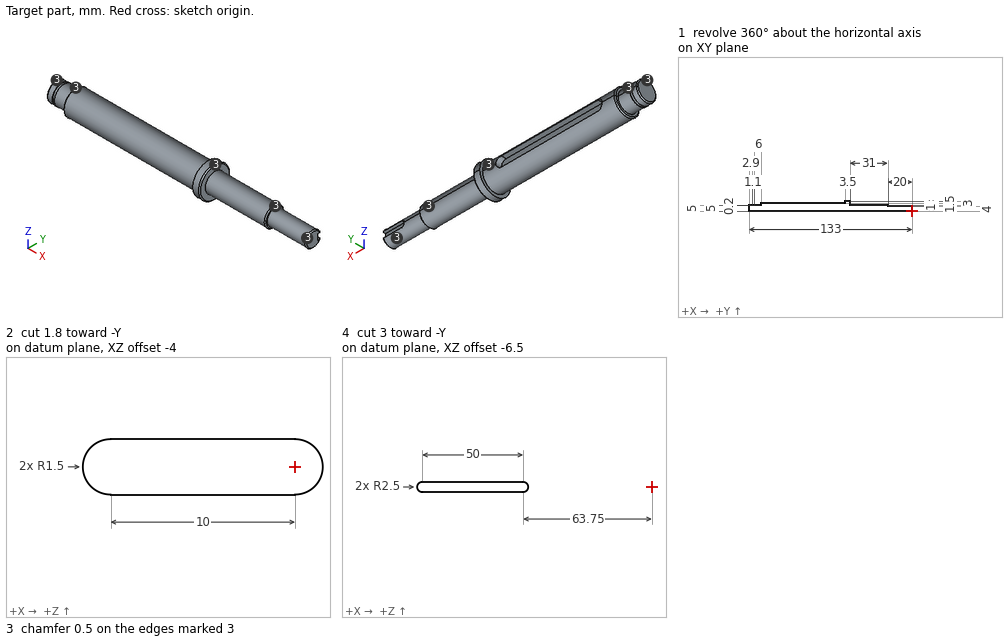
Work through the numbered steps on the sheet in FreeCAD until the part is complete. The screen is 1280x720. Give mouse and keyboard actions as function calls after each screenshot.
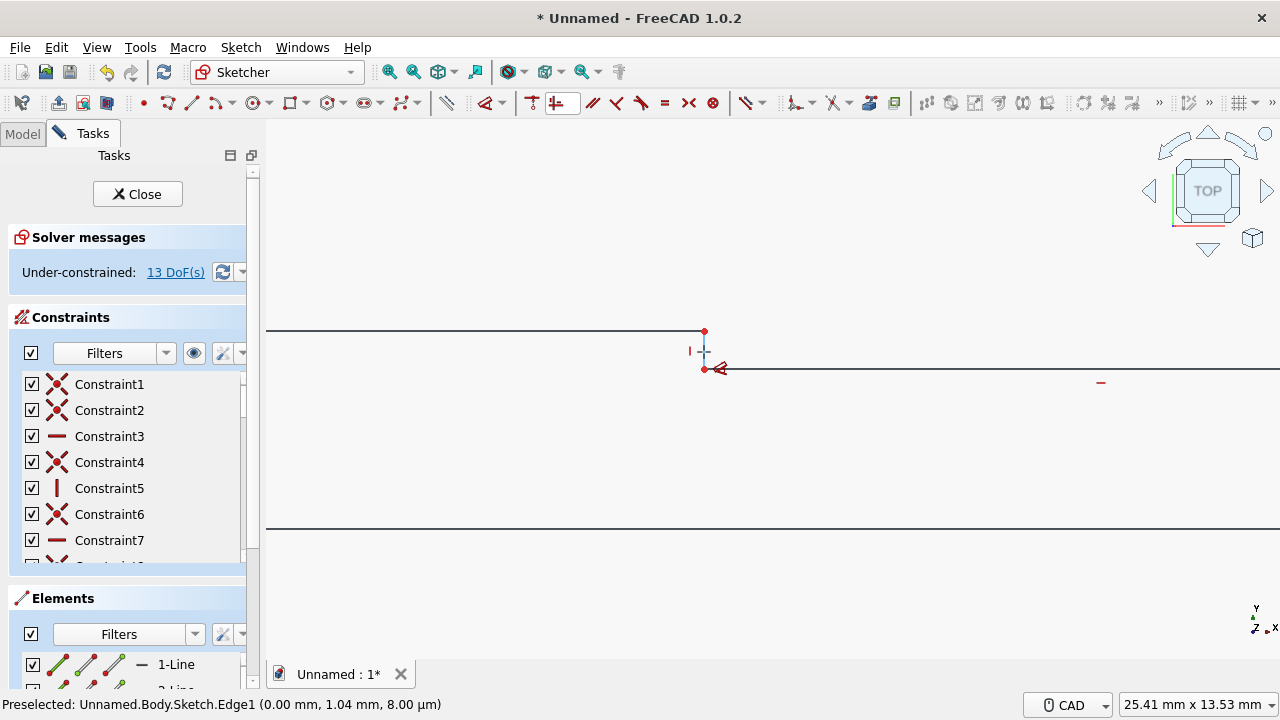
click(704, 350)
click(738, 350)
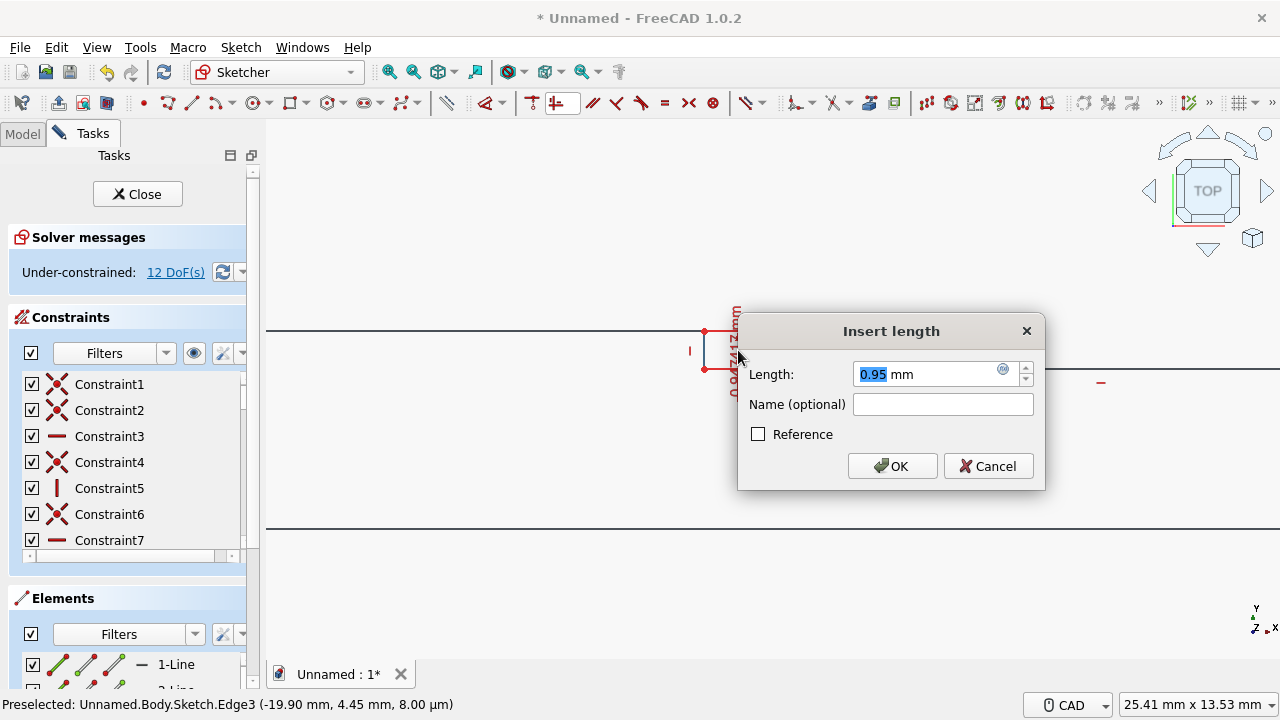
text(1)
key(Return)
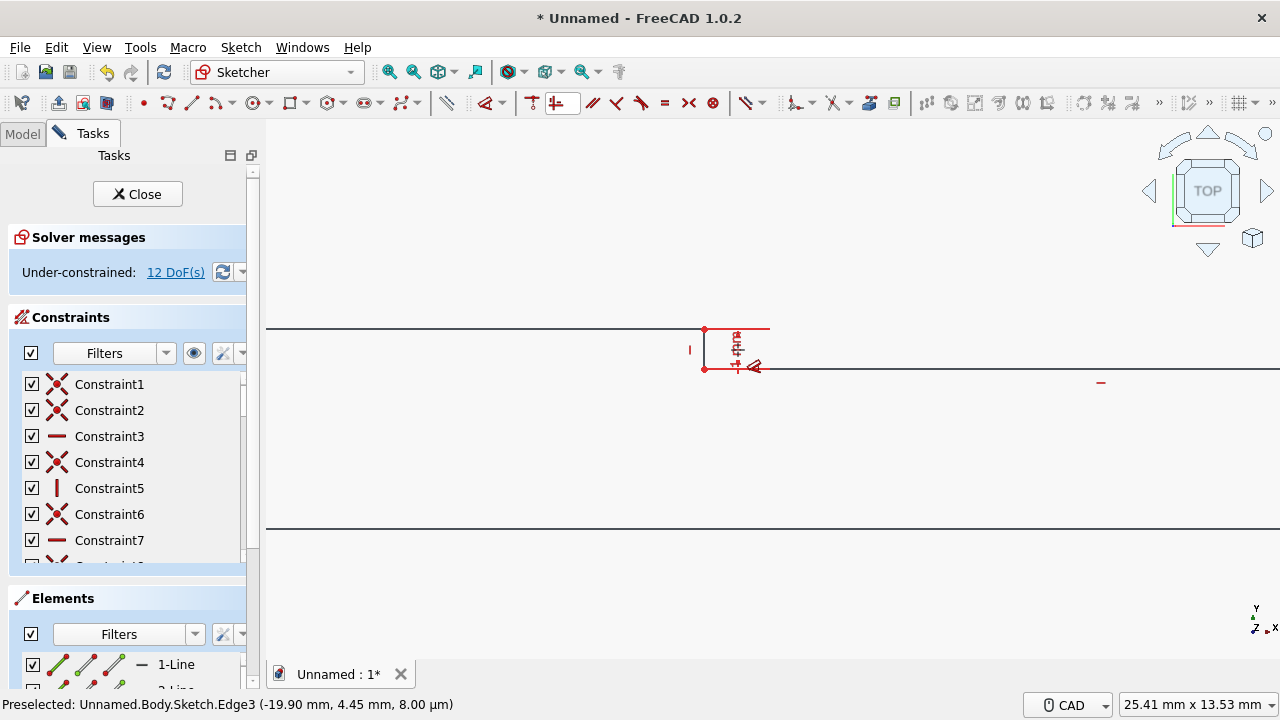
scroll(936, 391, down, 11)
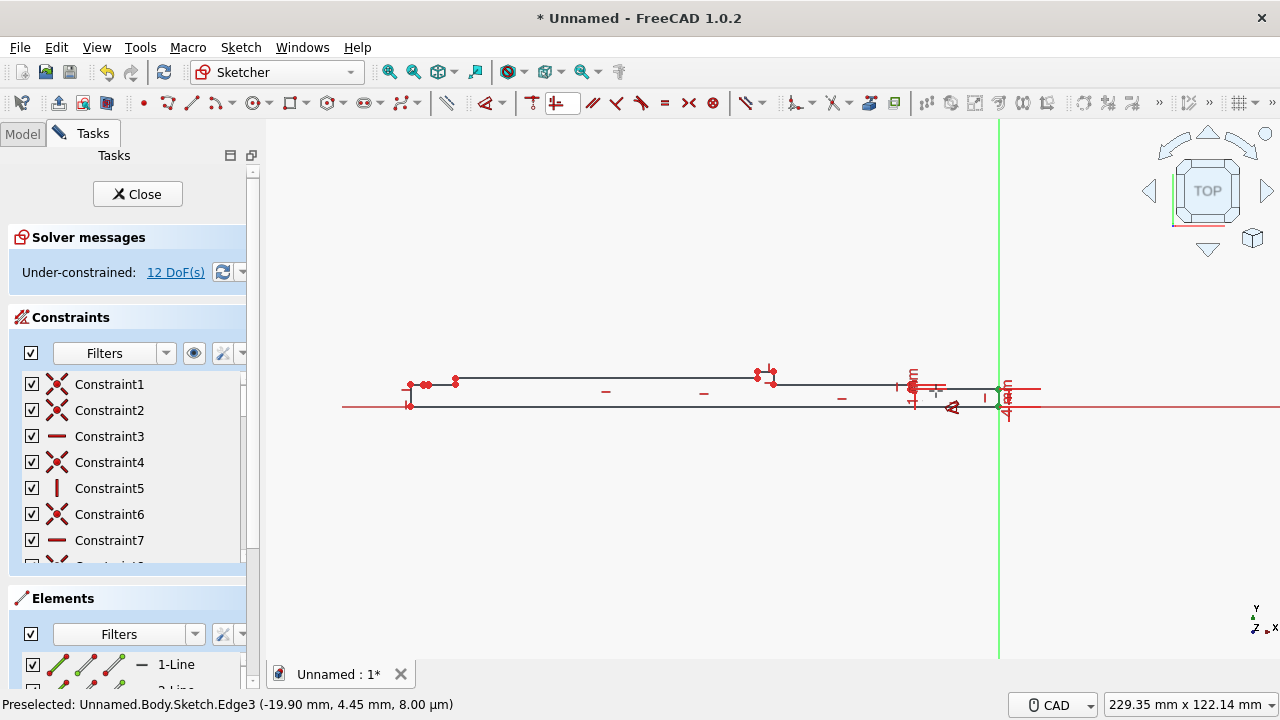
scroll(774, 381, up, 7)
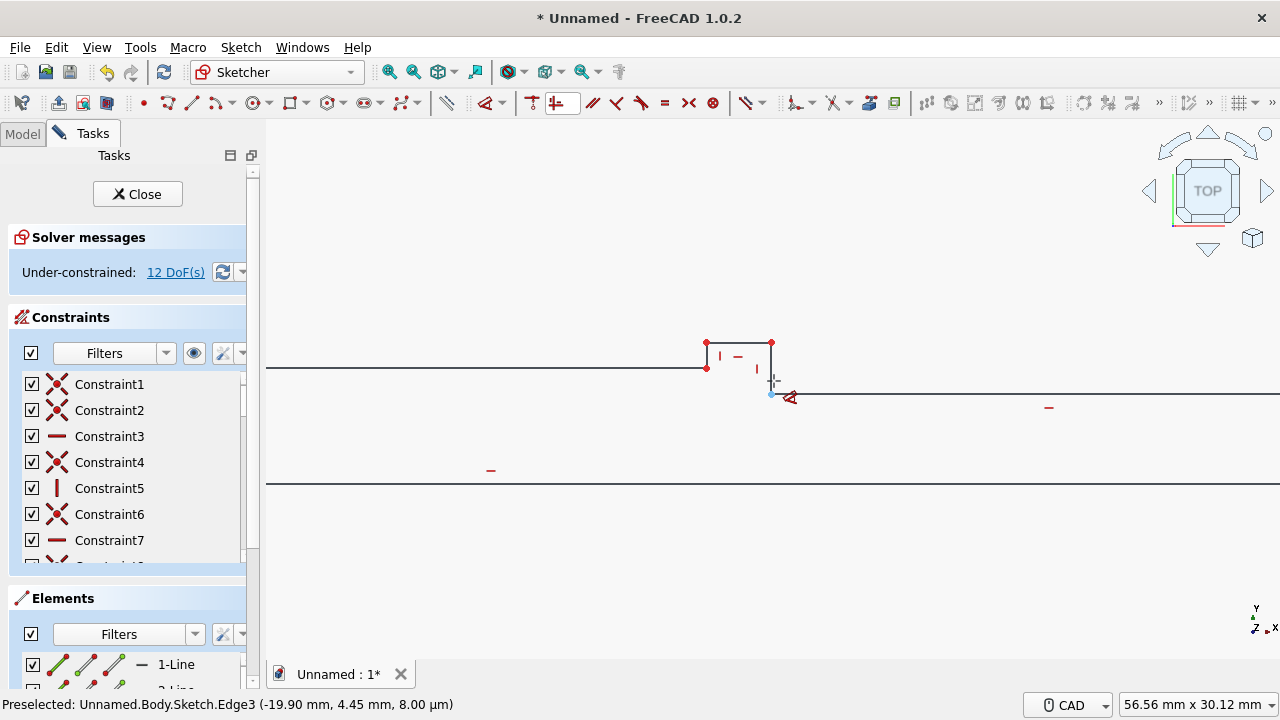
click(771, 379)
click(805, 368)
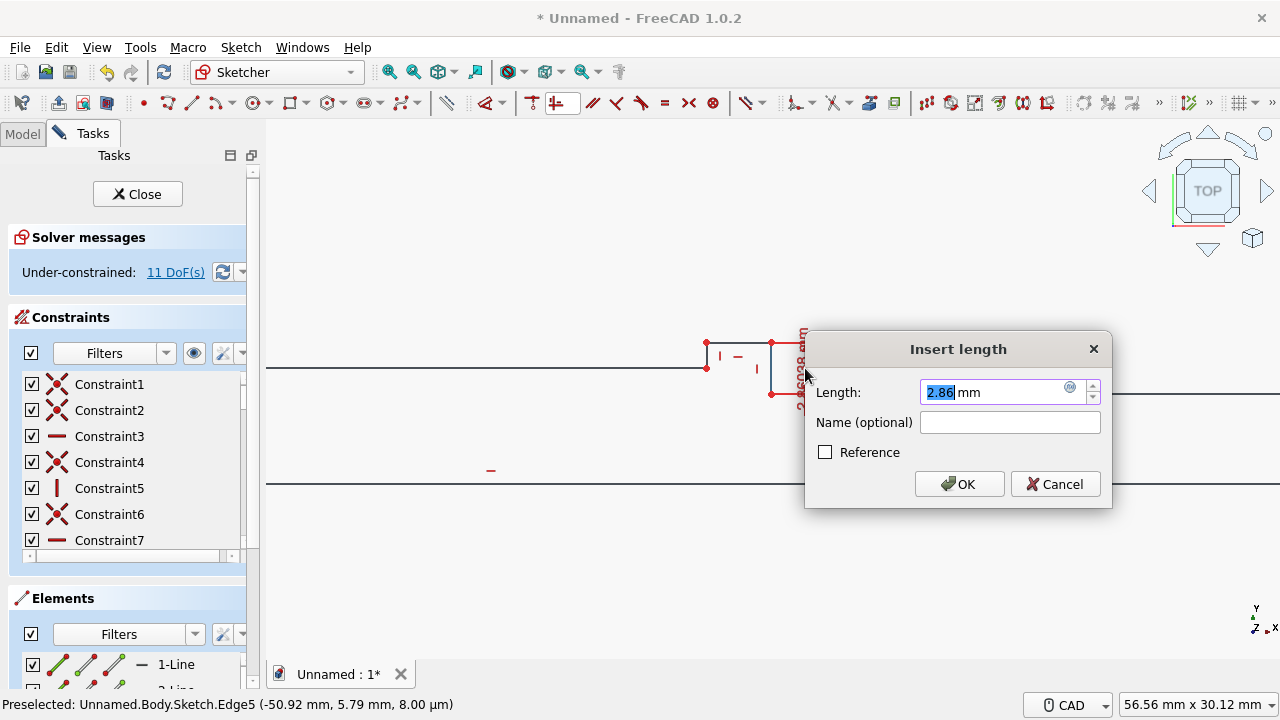
text(3)
key(Return)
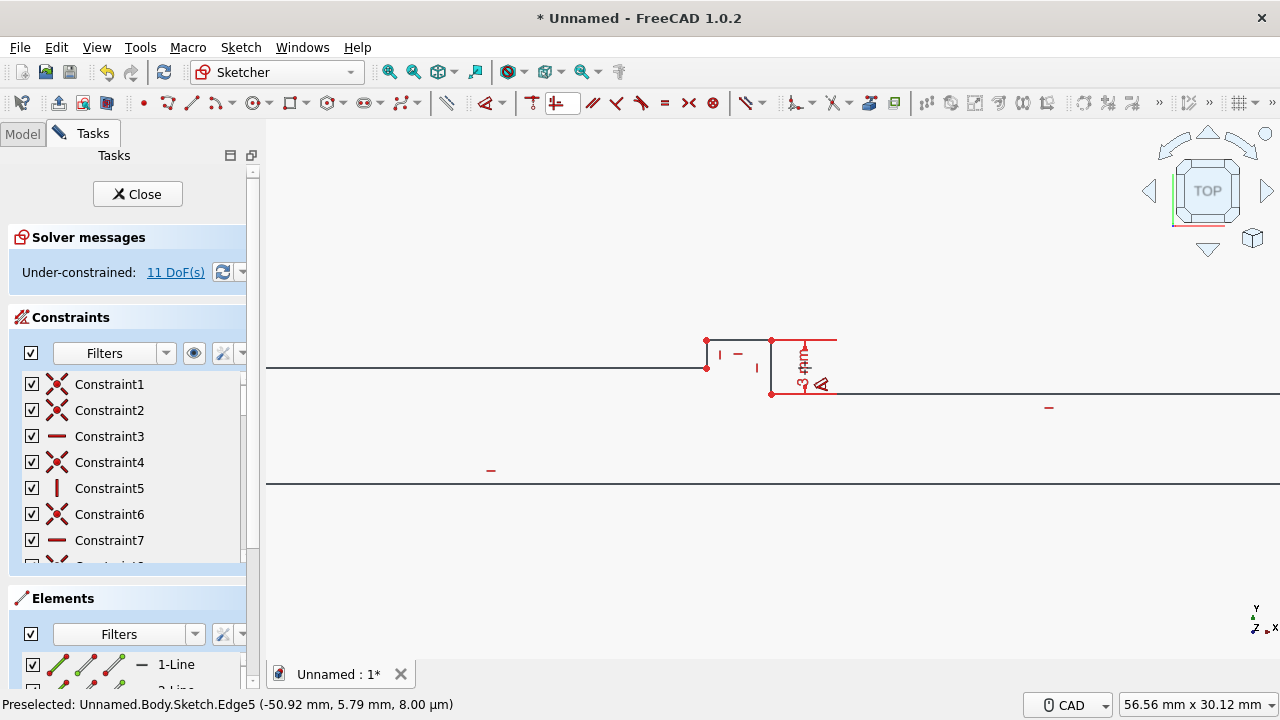
scroll(774, 381, down, 7)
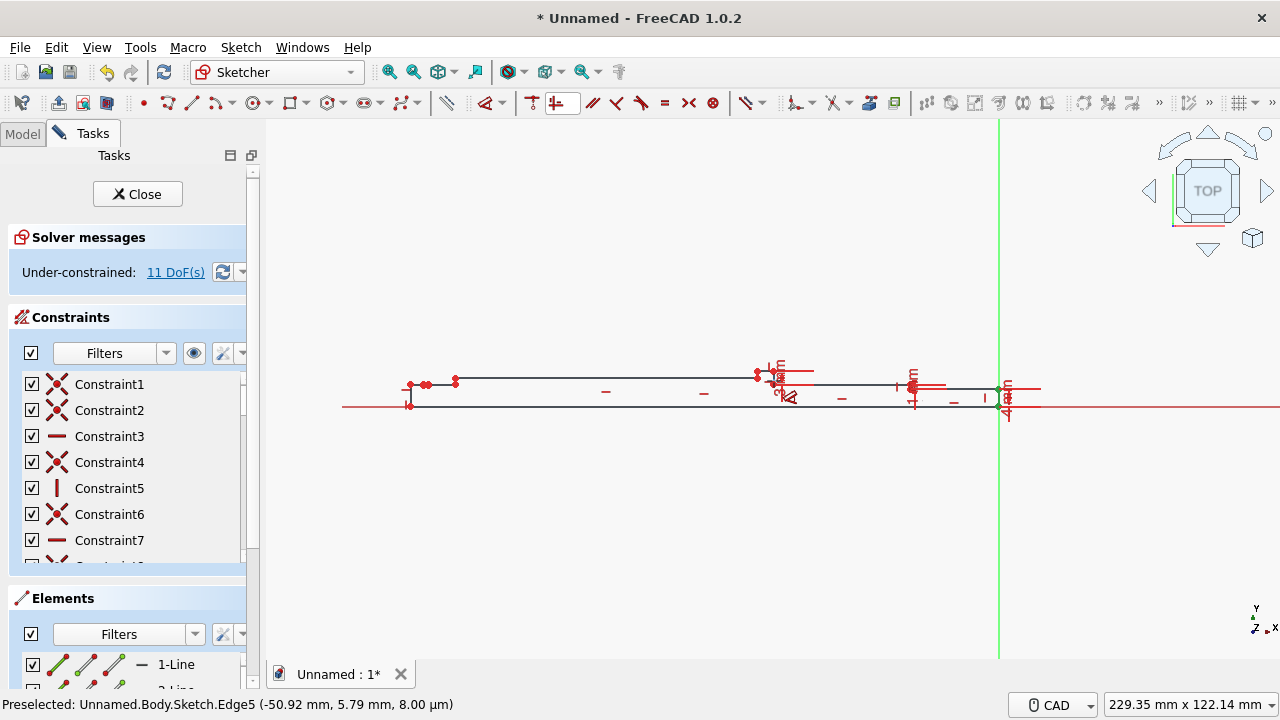
scroll(447, 385, up, 3)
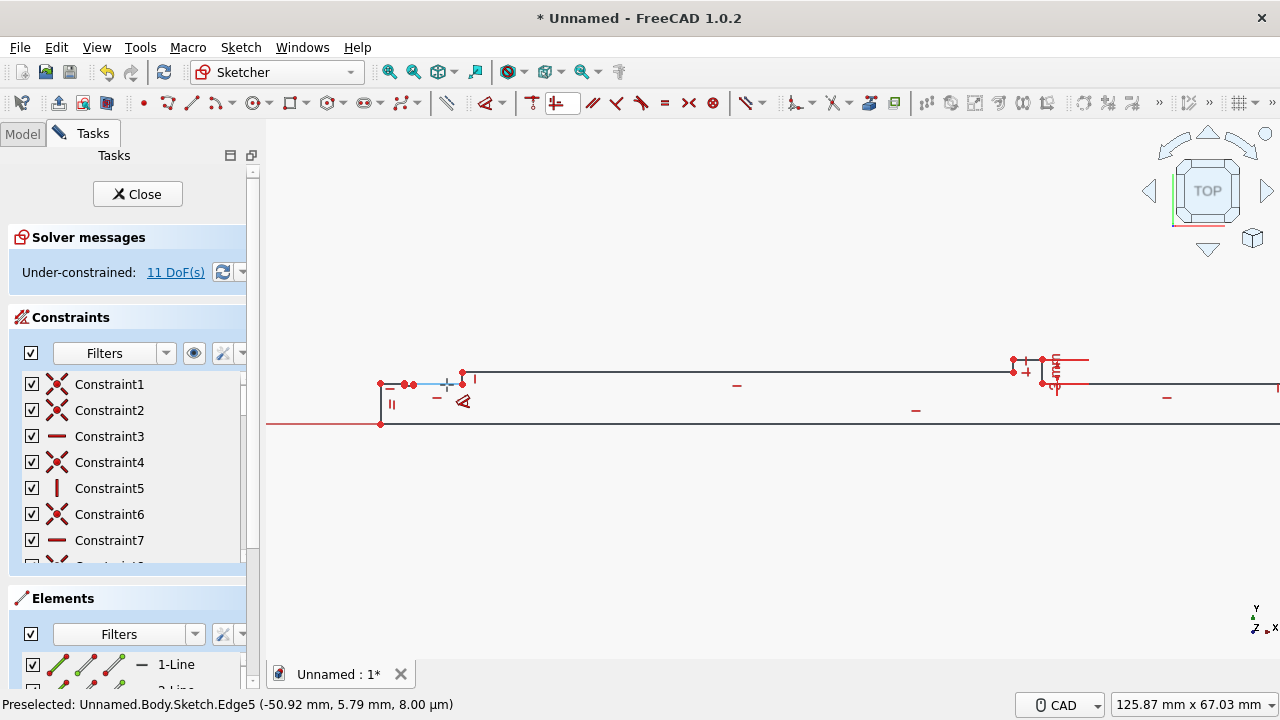
click(448, 384)
click(438, 350)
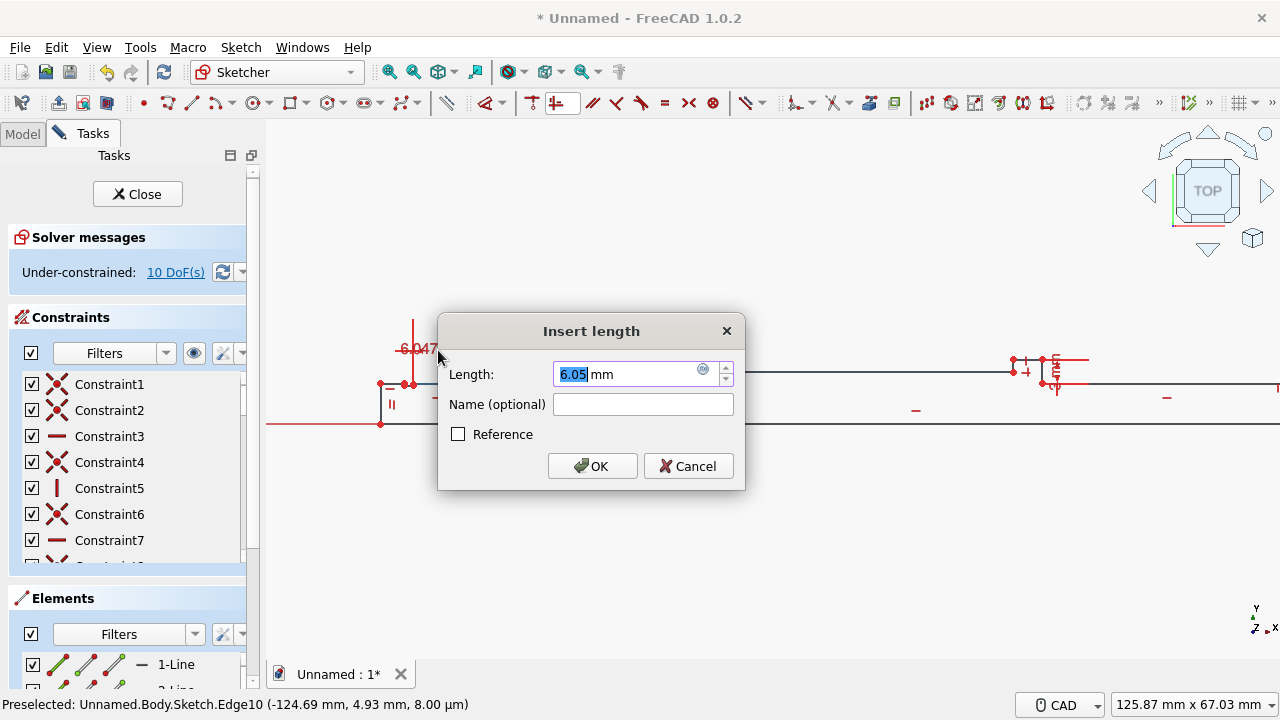
text(6)
key(Return)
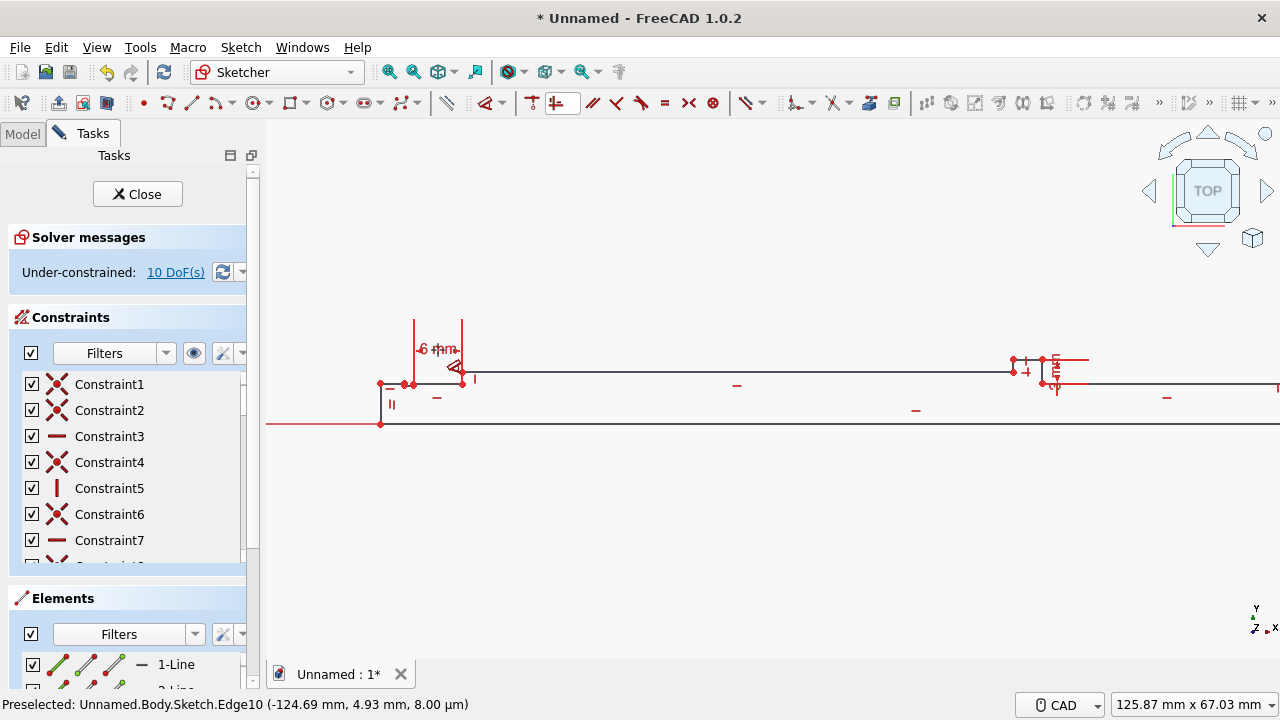
click(381, 396)
click(347, 404)